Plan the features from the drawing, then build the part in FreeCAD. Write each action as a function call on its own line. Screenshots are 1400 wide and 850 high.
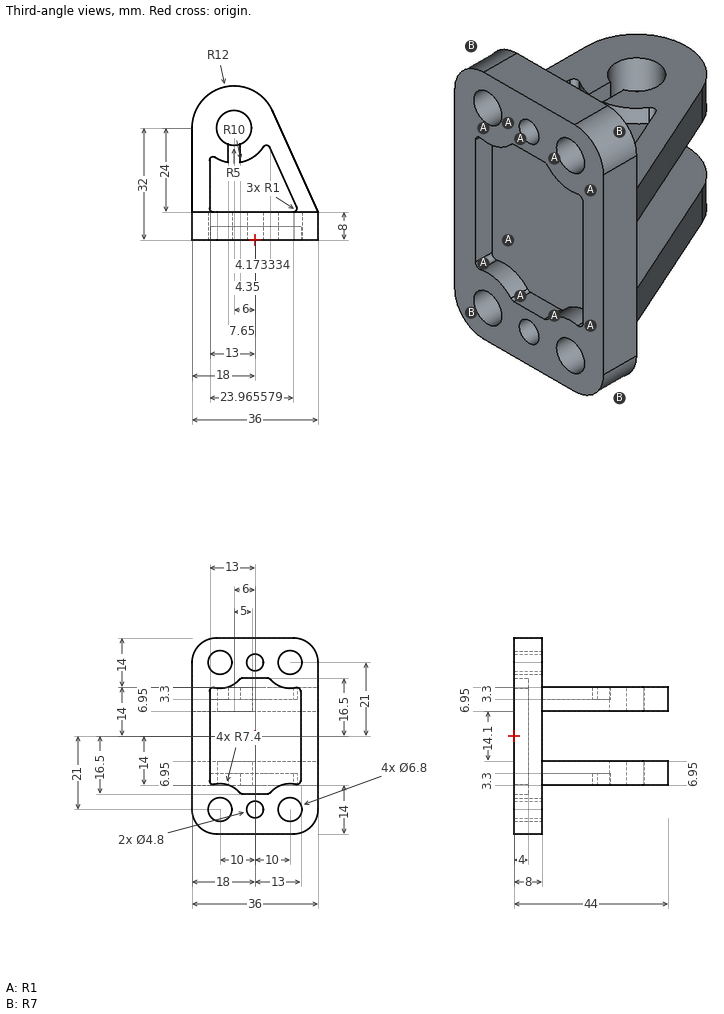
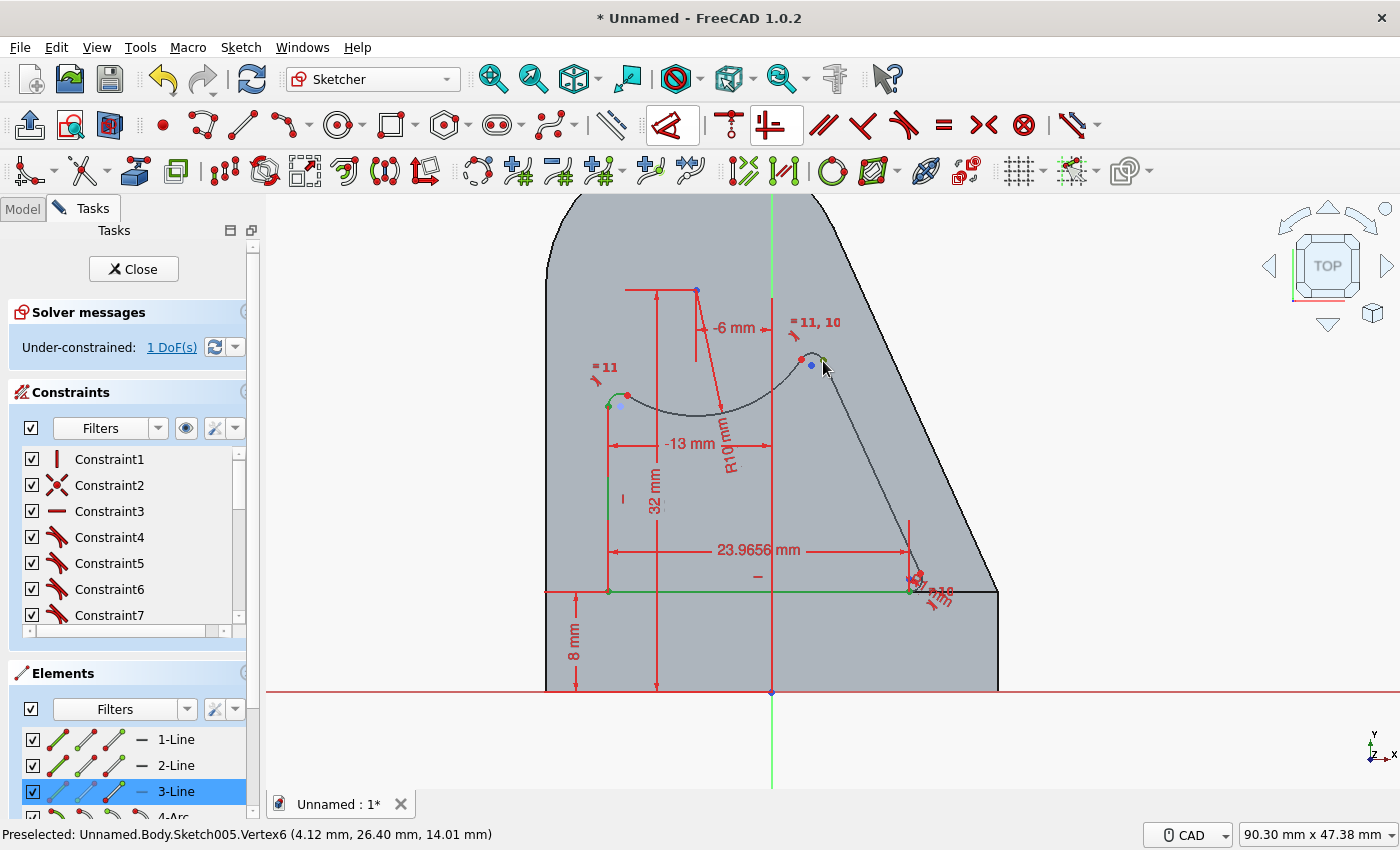
click(694, 126)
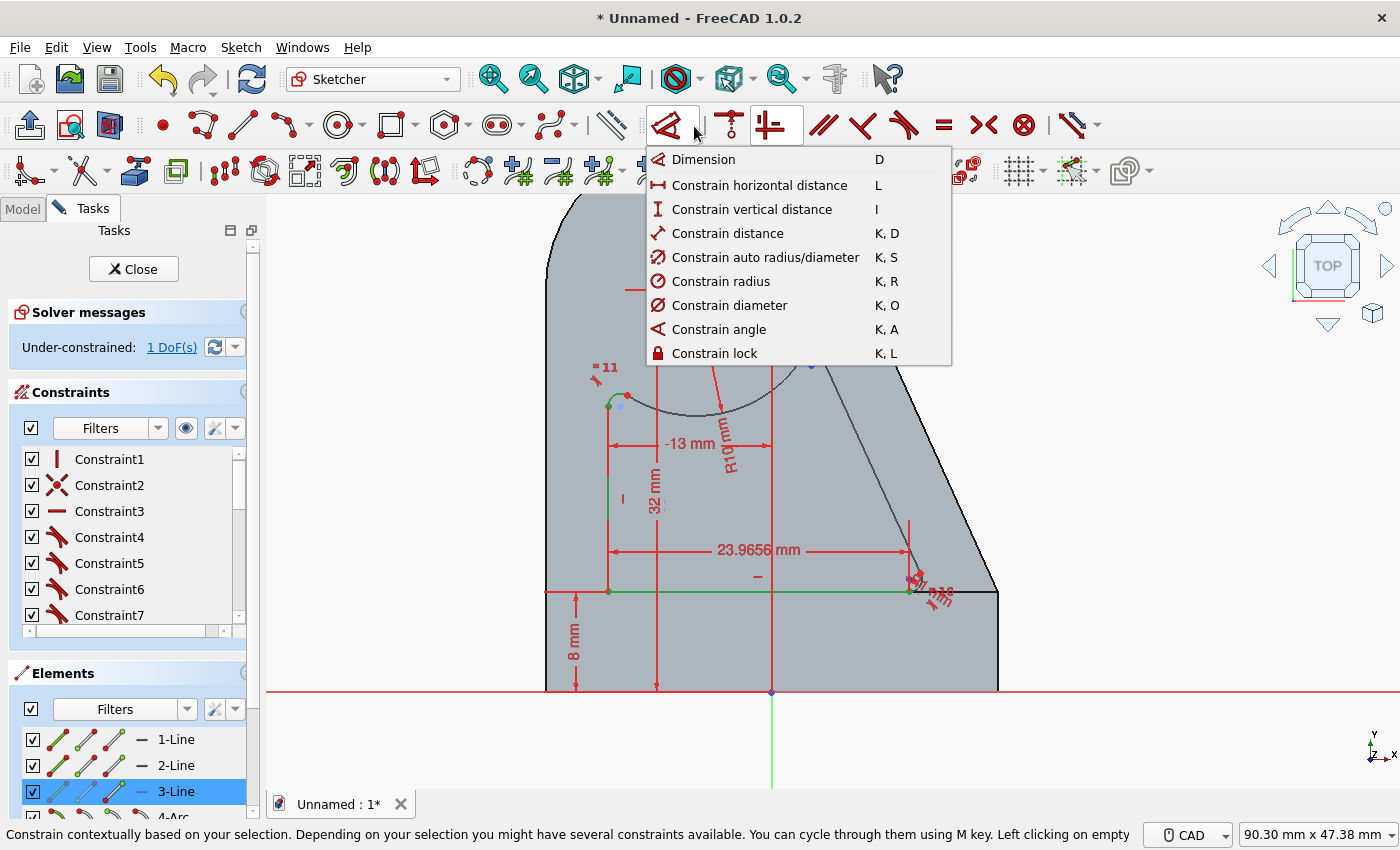
click(799, 185)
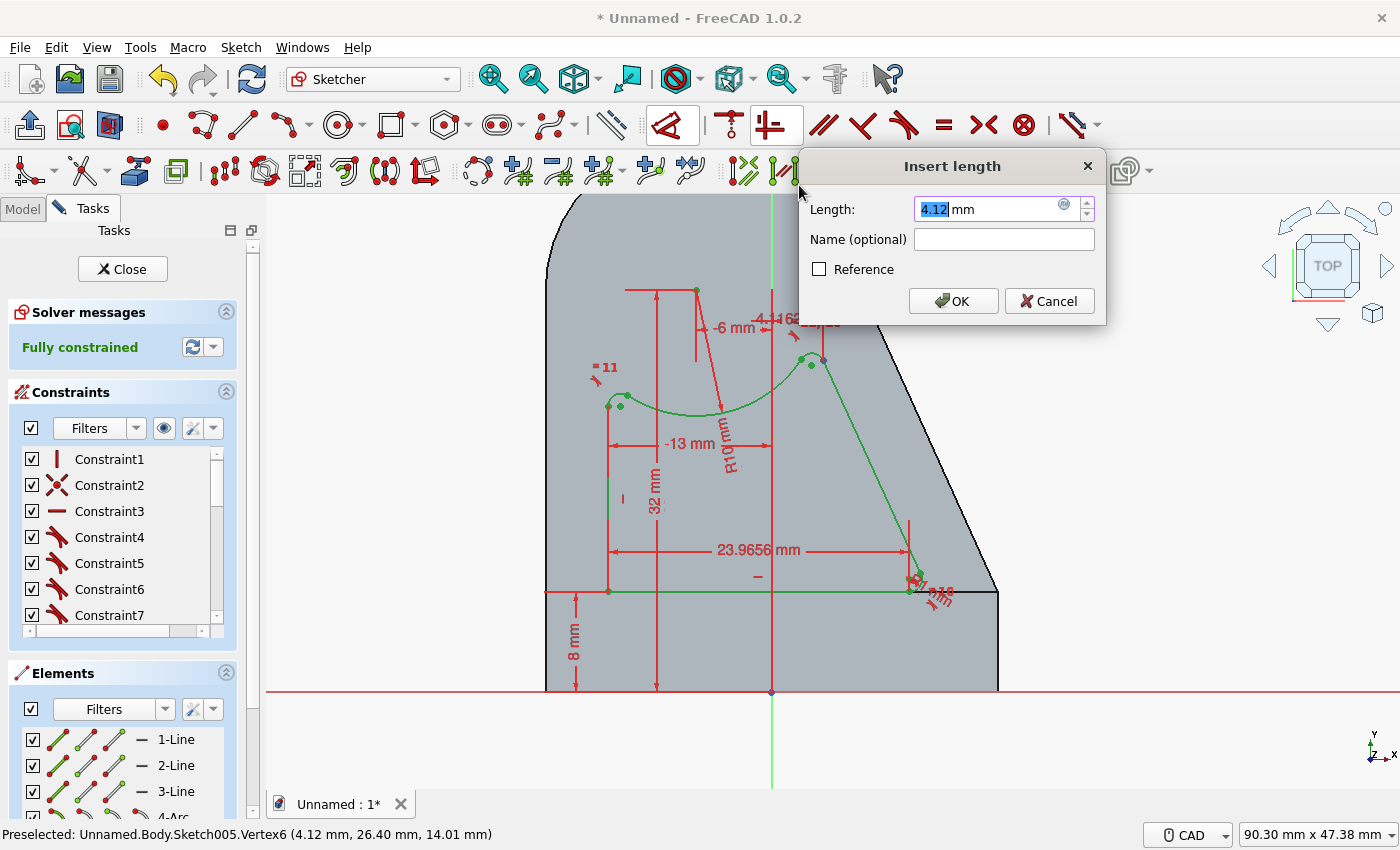
text(4.173334)
key(Return)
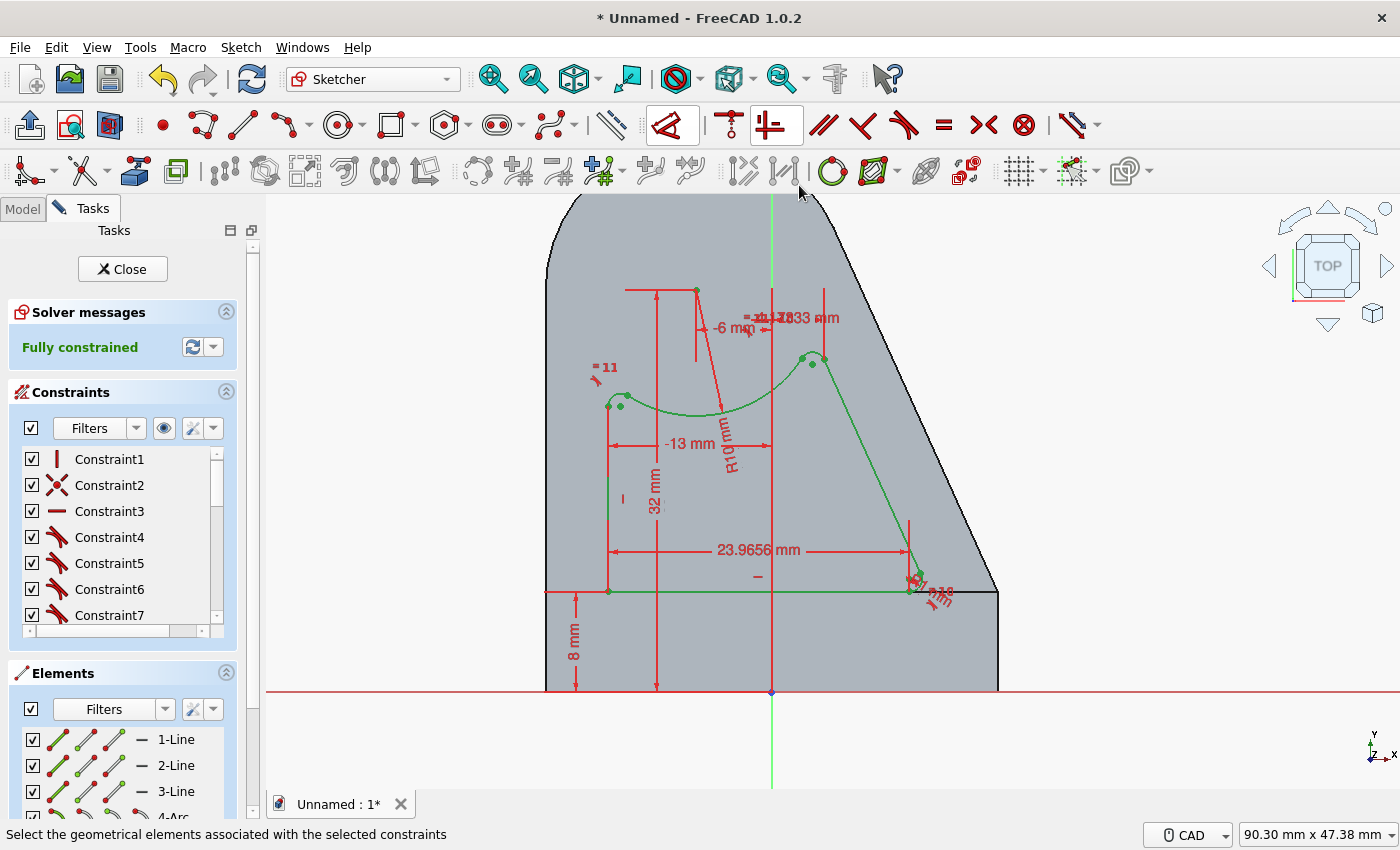
click(123, 269)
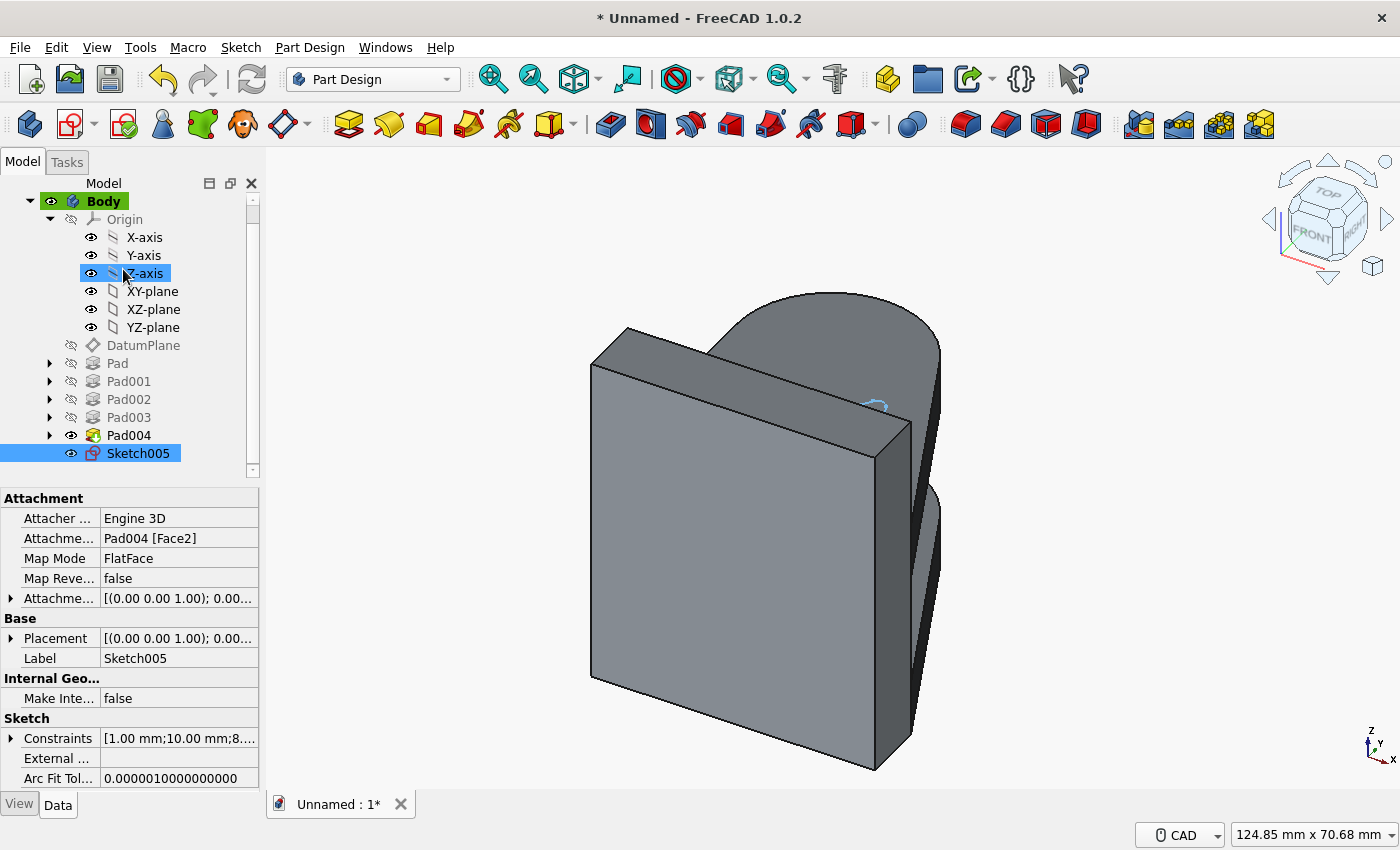
click(612, 124)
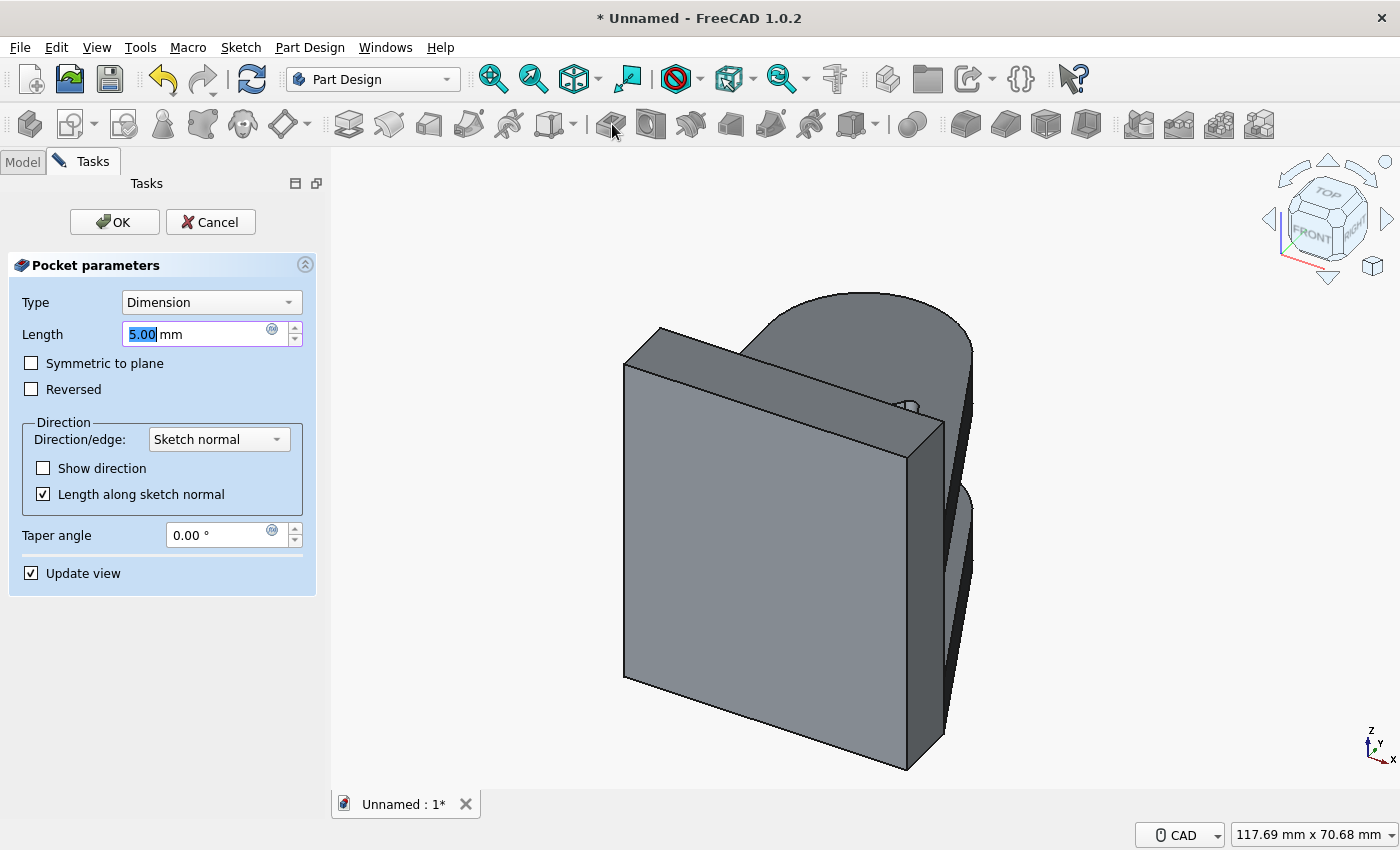
text(3.3)
key(Tab)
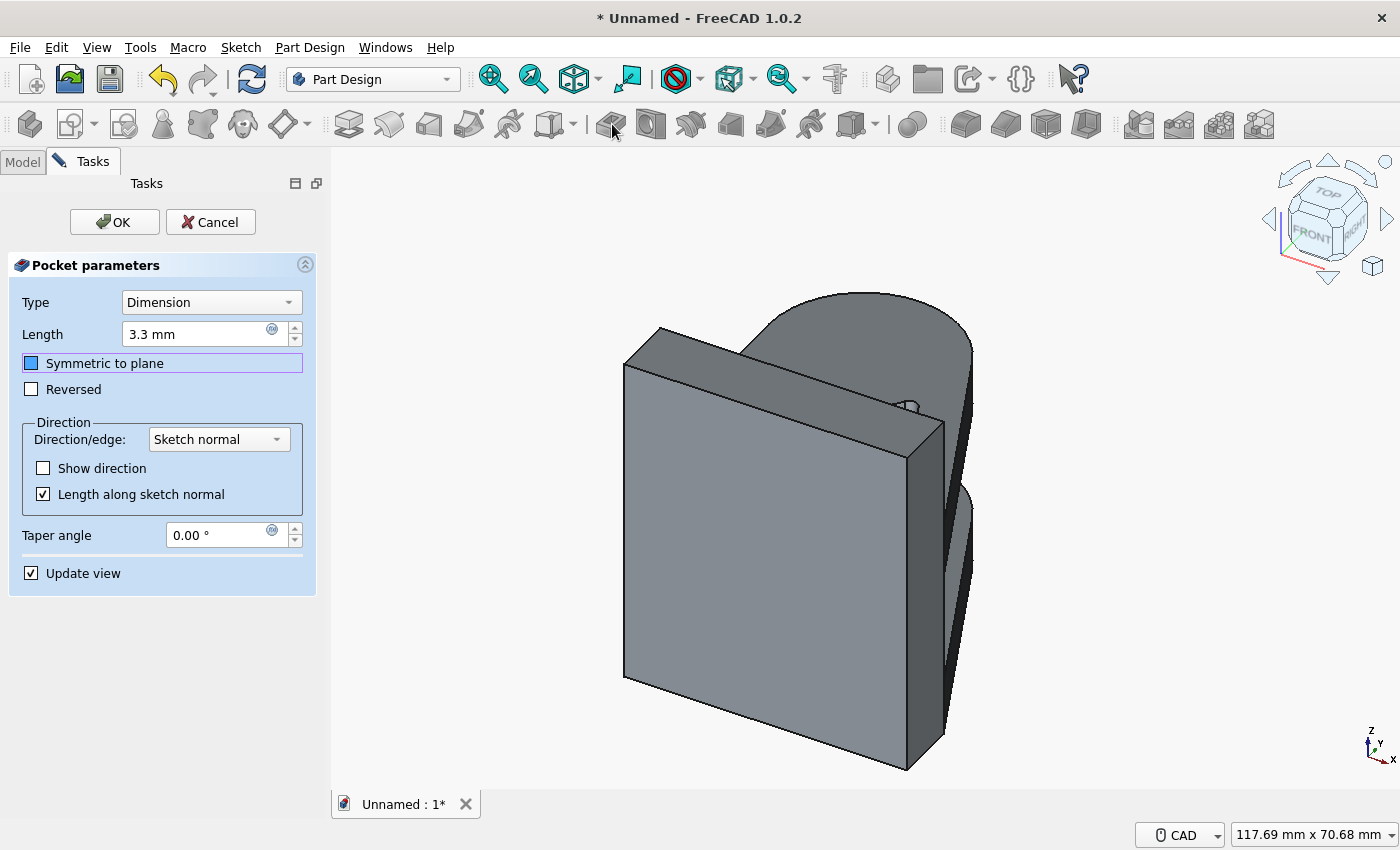
click(115, 222)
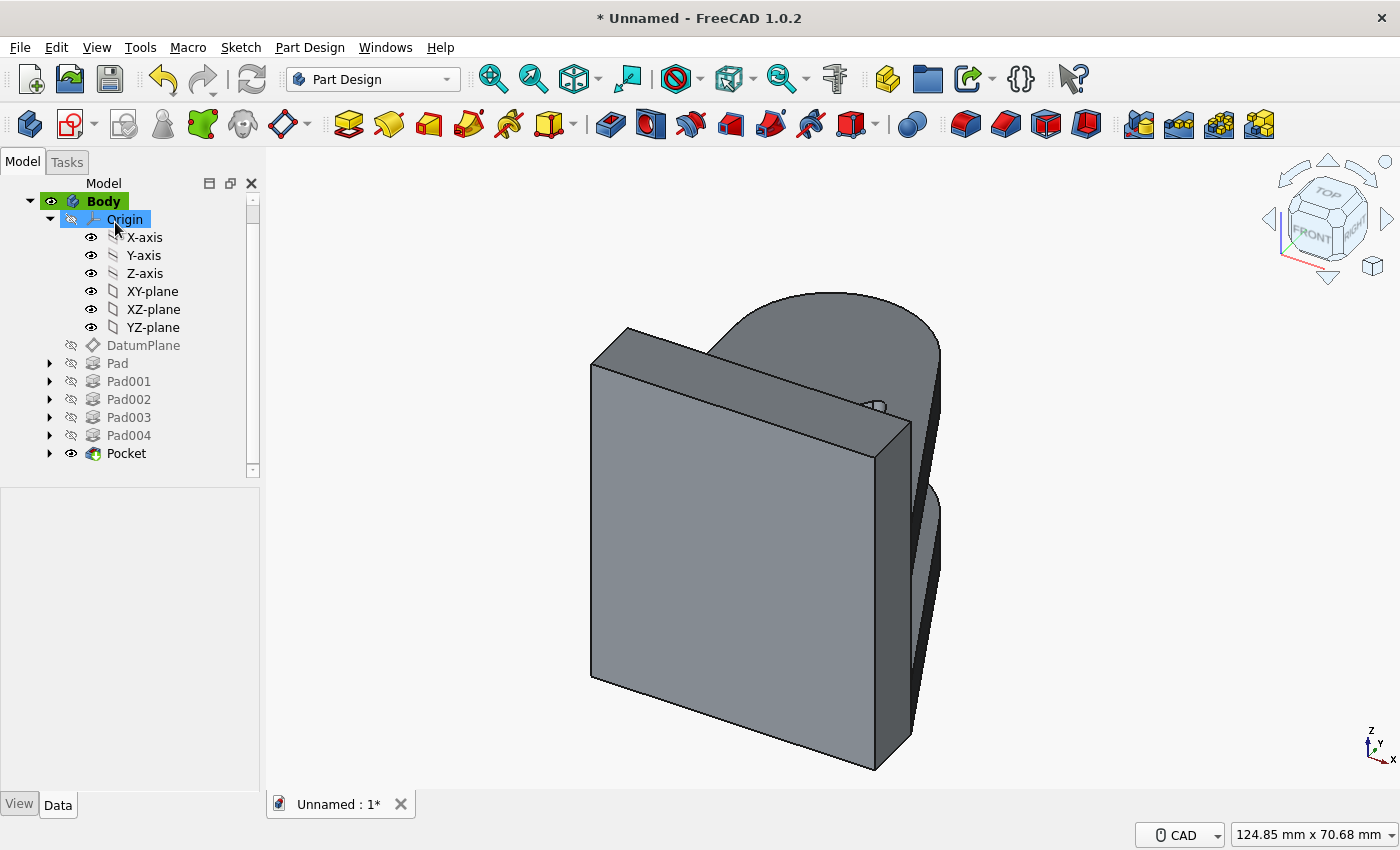
key(5)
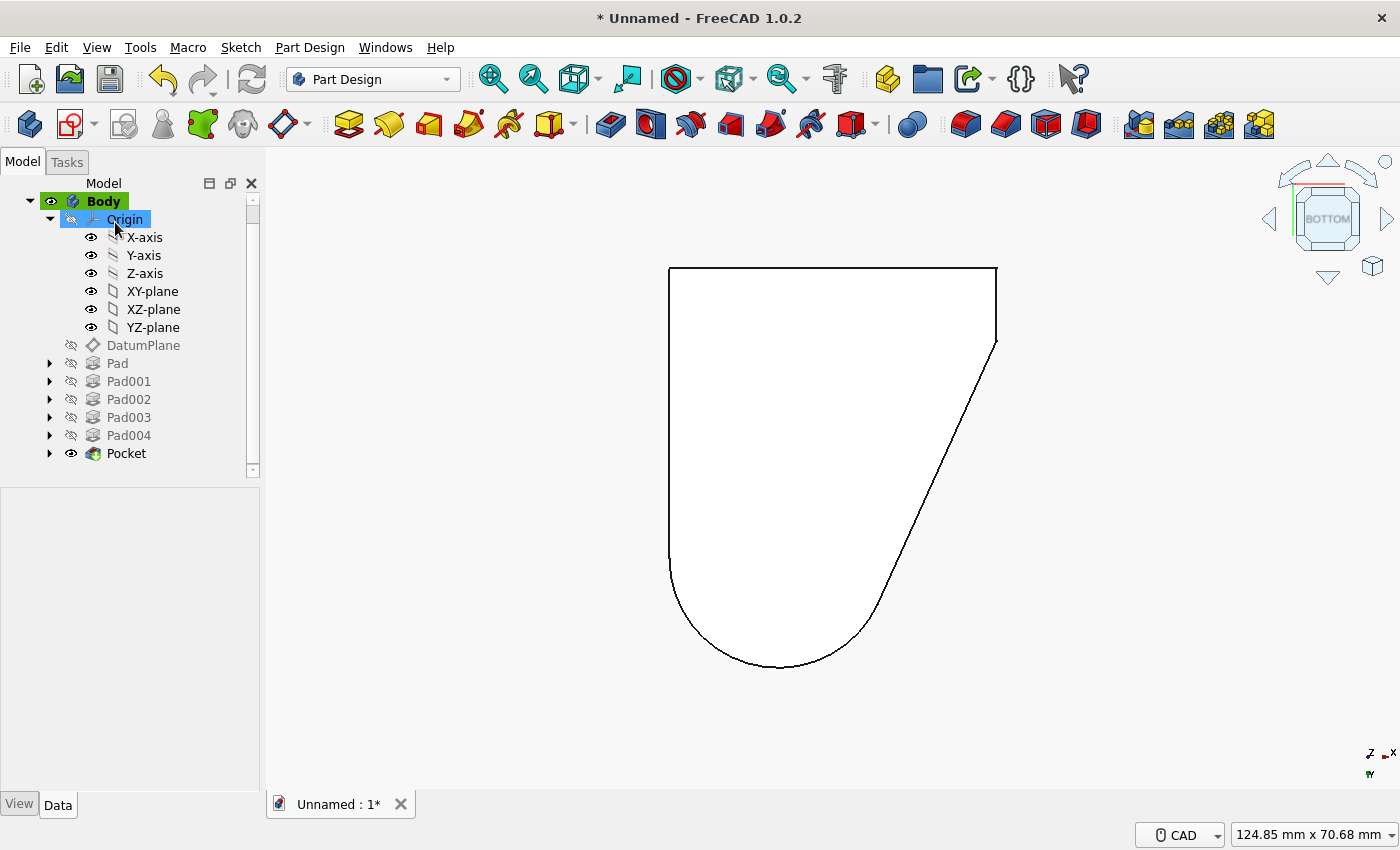
click(833, 410)